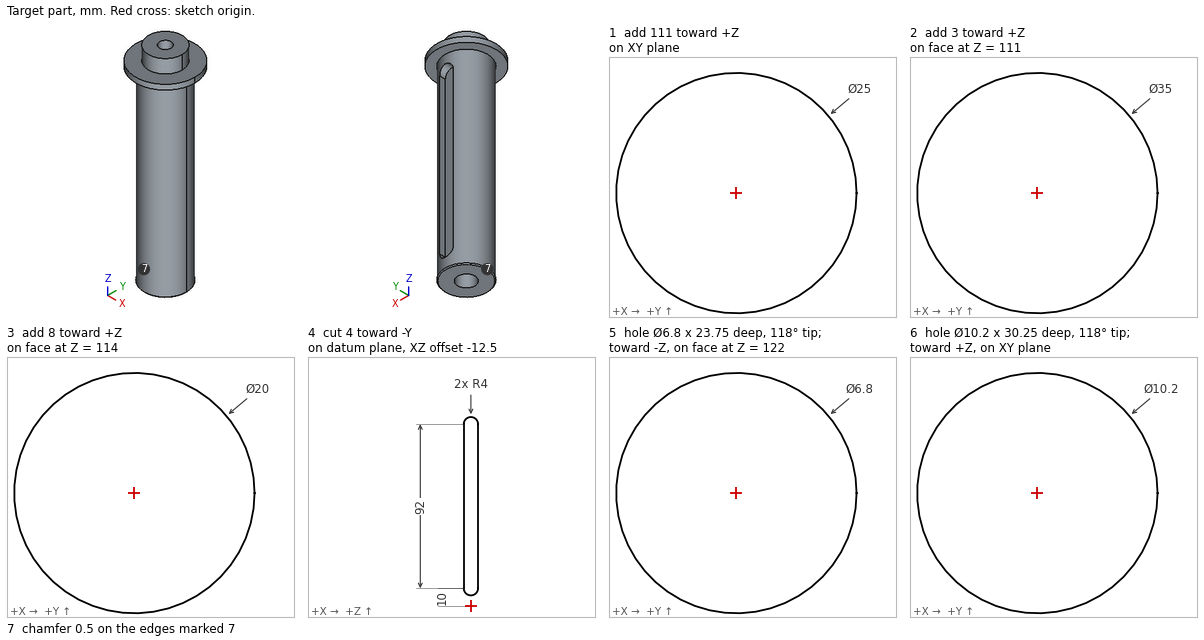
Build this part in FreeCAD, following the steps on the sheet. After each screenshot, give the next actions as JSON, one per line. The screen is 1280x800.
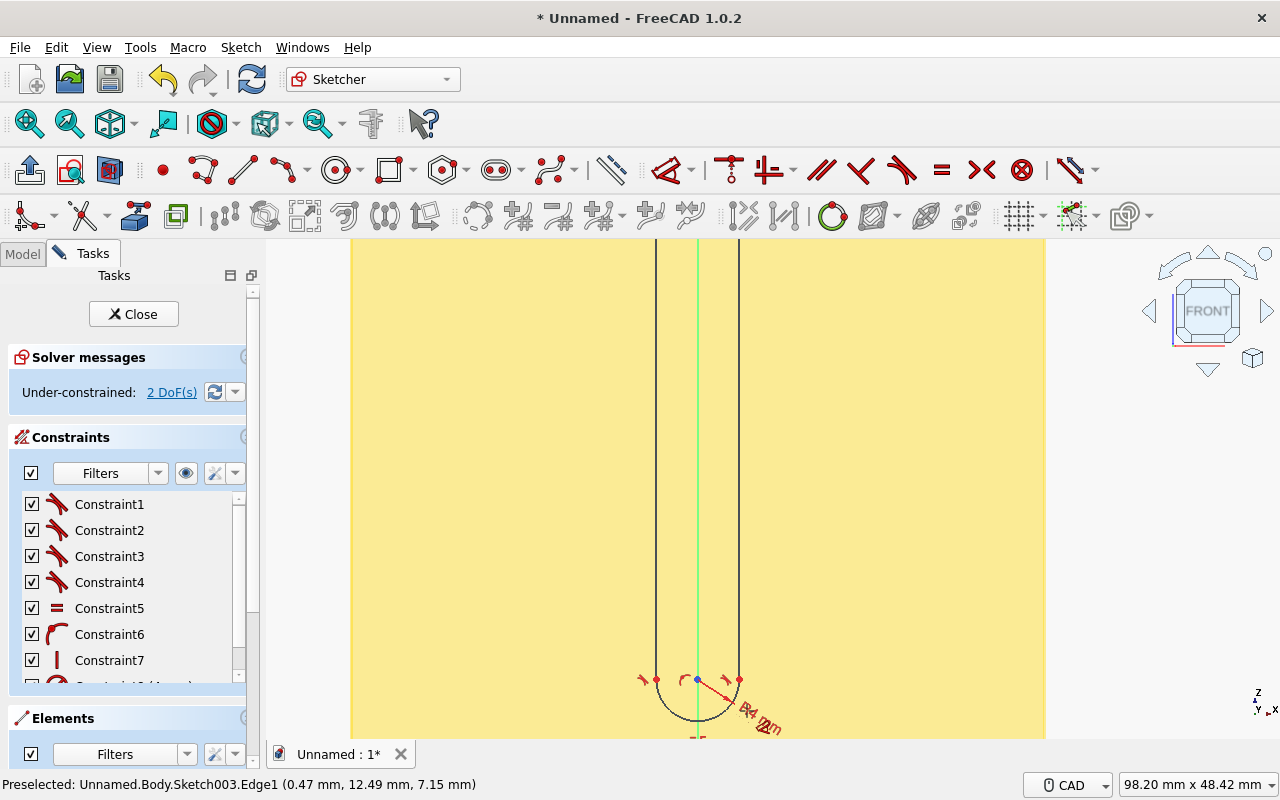
{"action": "left_click", "coordinate": [656, 395]}
{"action": "left_click", "coordinate": [622, 473]}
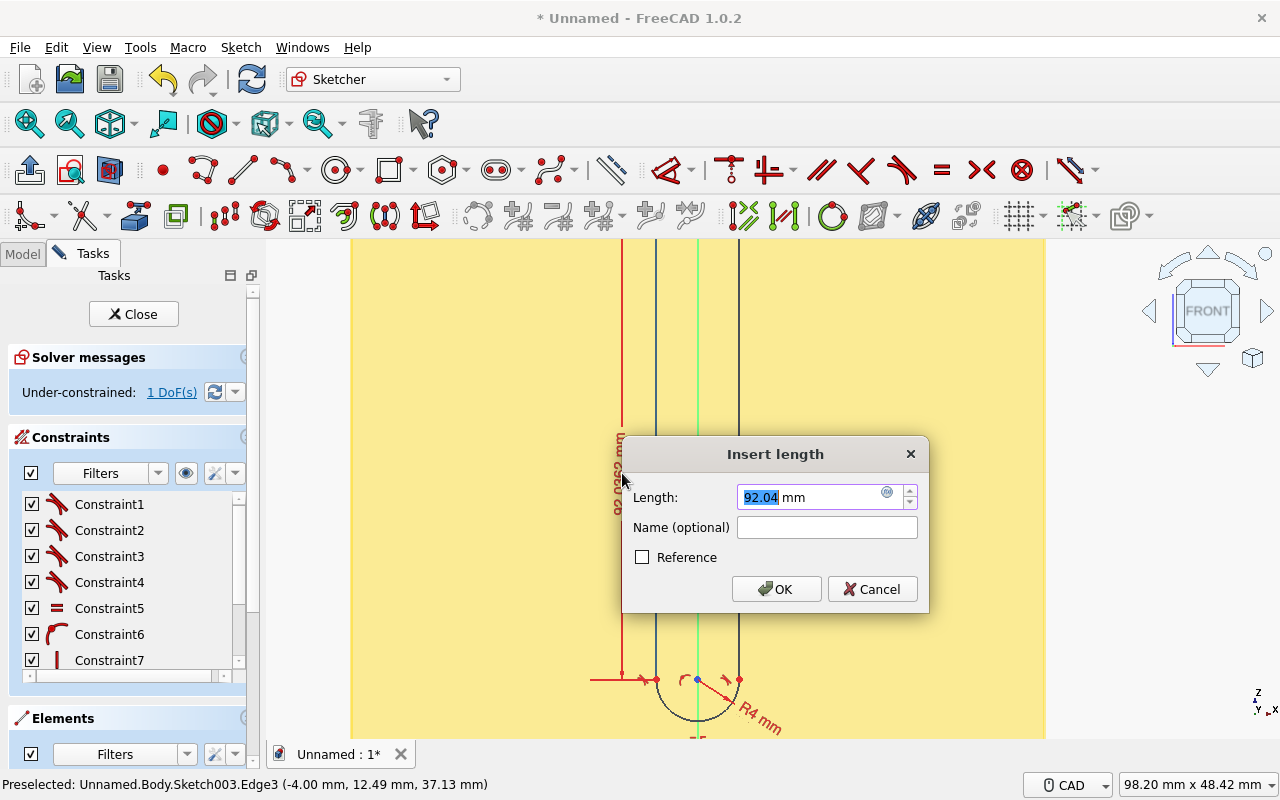
{"action": "type", "text": "92"}
{"action": "key", "text": "Return"}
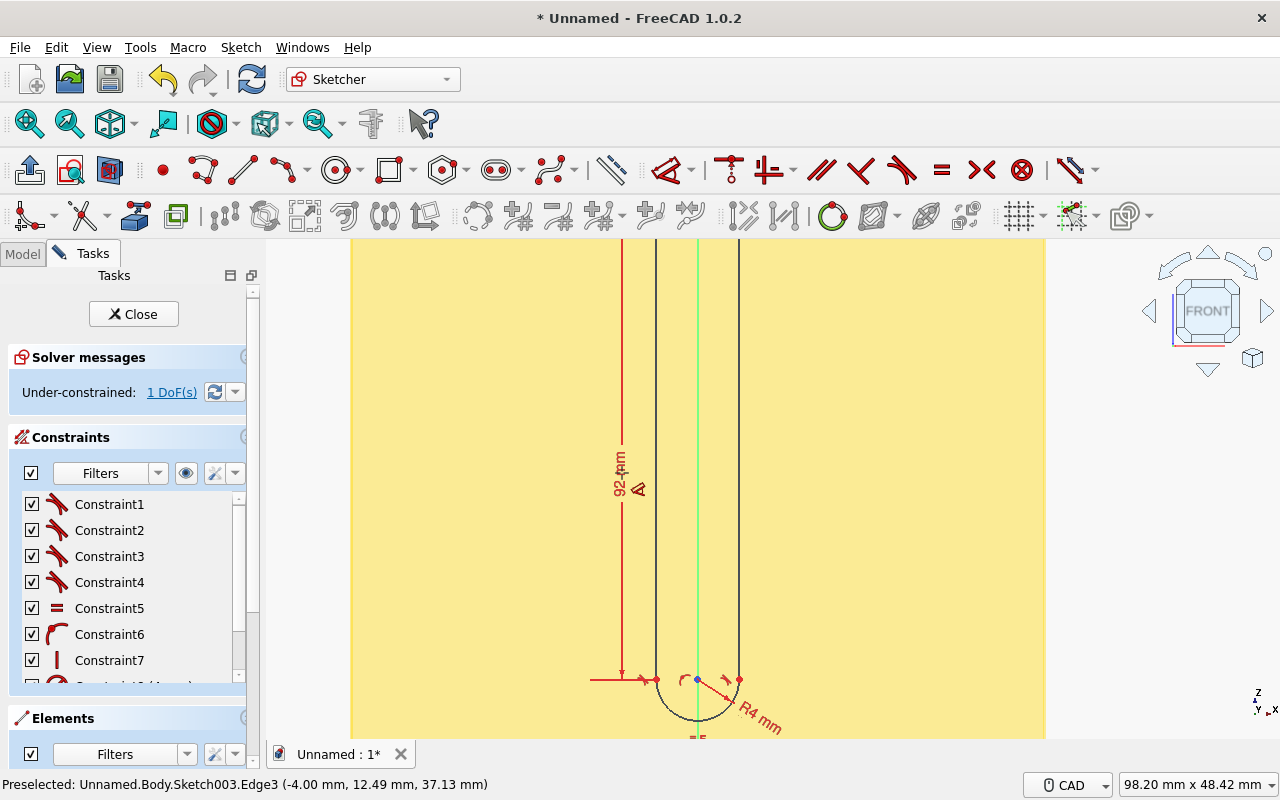
{"action": "left_click", "coordinate": [656, 680]}
{"action": "left_click", "coordinate": [622, 695]}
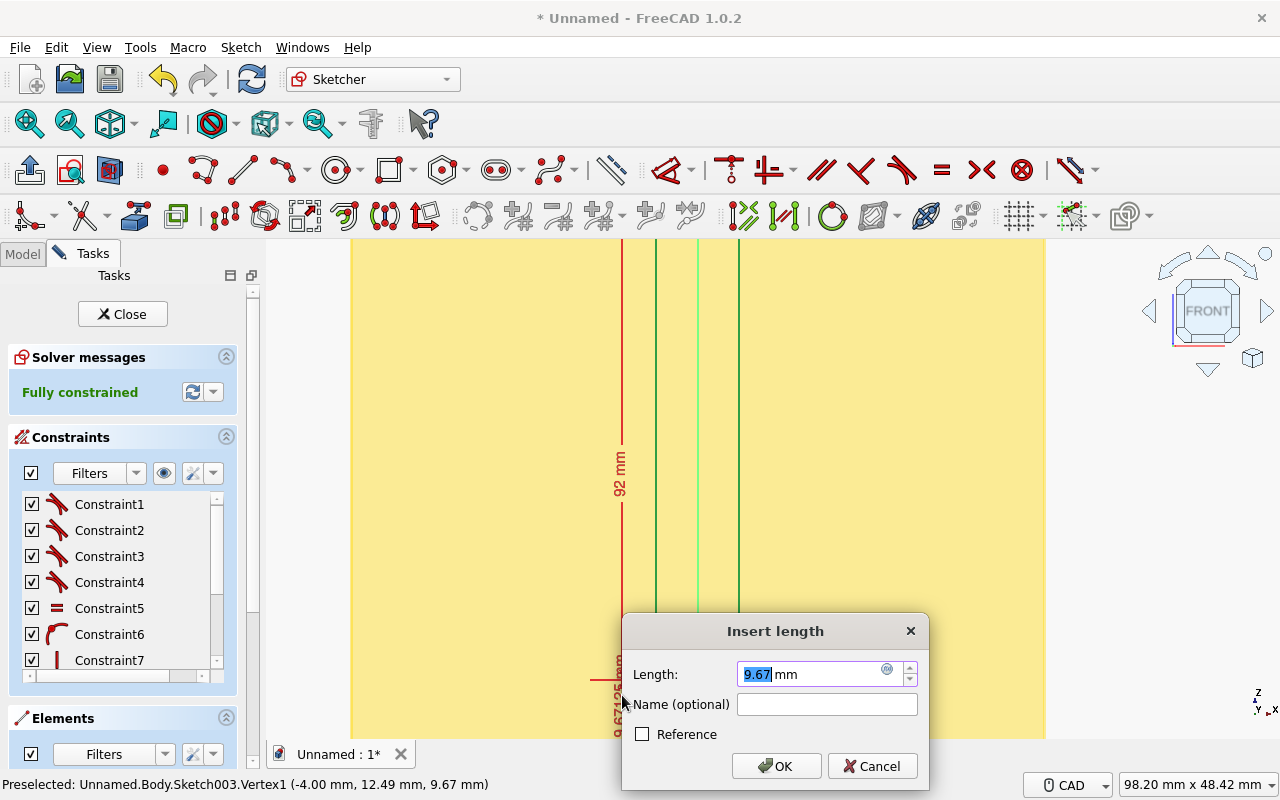
{"action": "type", "text": "10"}
{"action": "key", "text": "Return"}
{"action": "key", "text": "Escape"}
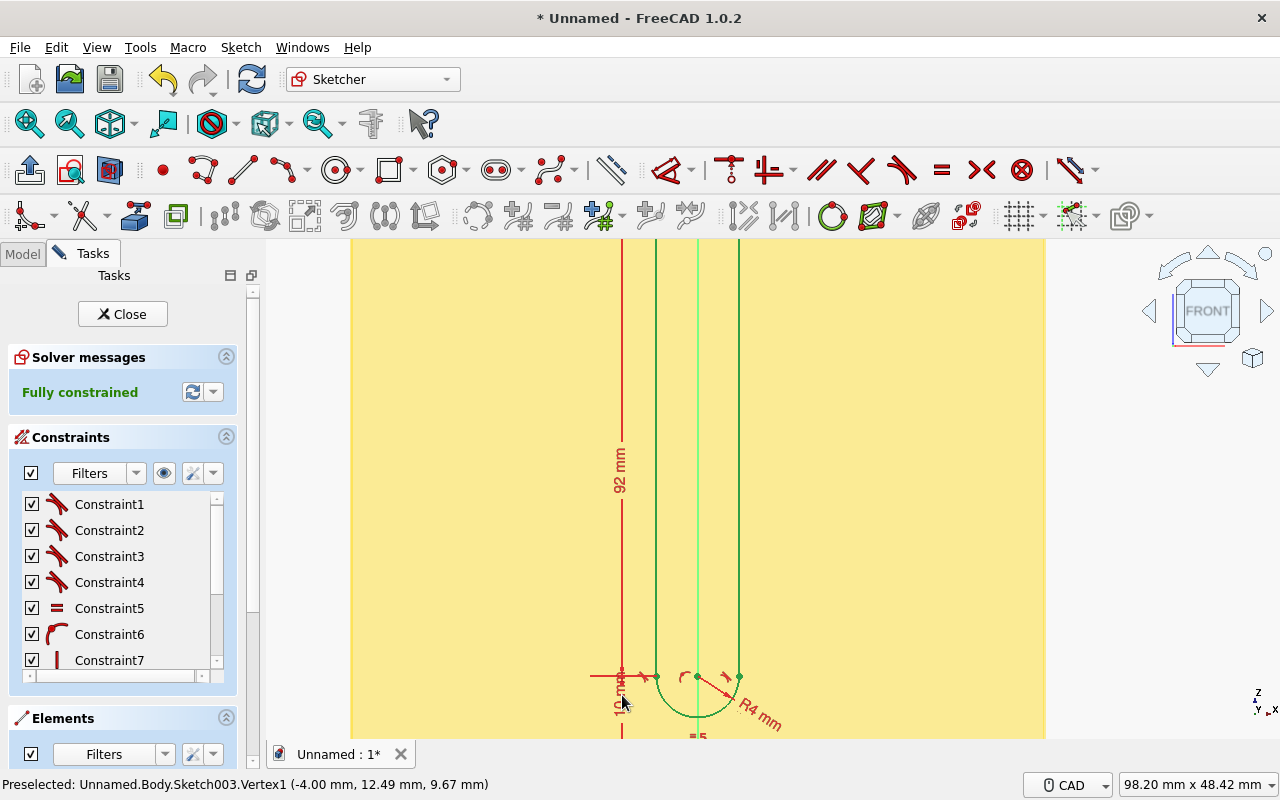
{"action": "left_click", "coordinate": [123, 314]}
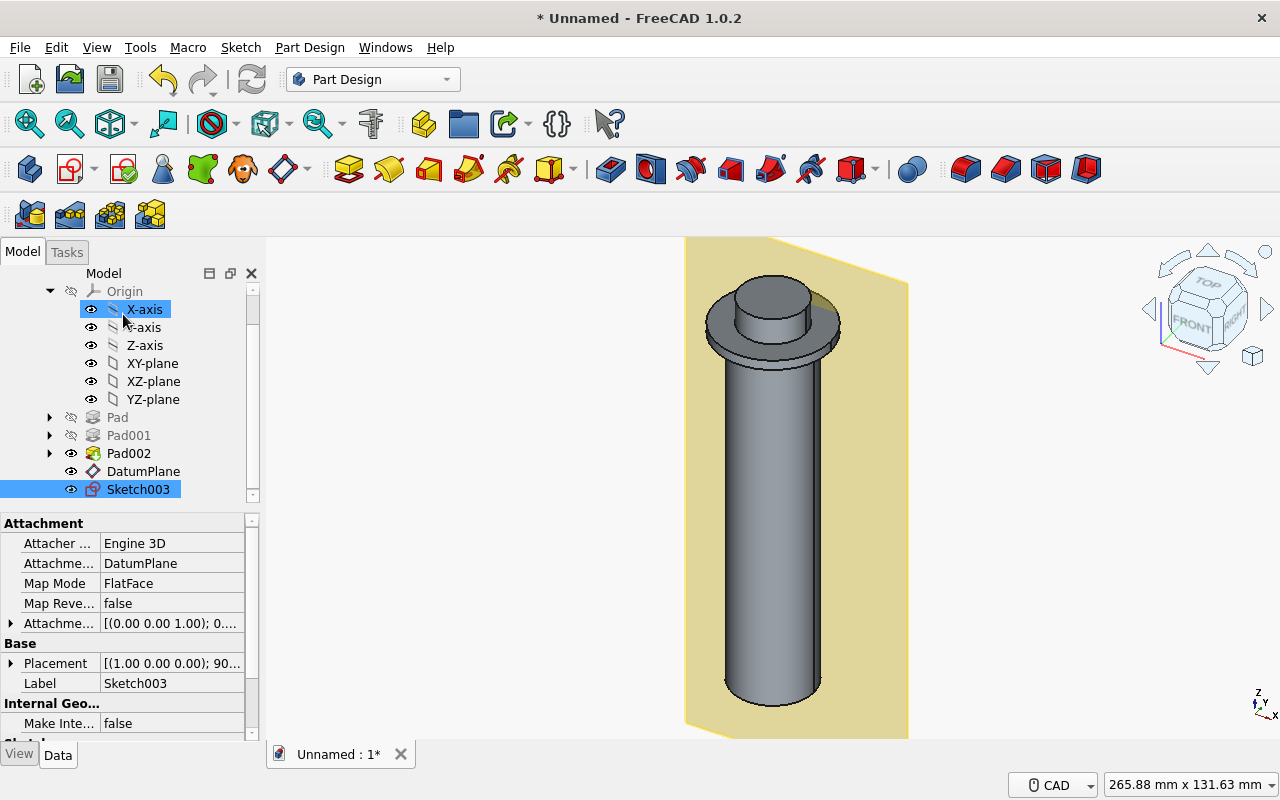
{"action": "left_click", "coordinate": [612, 170]}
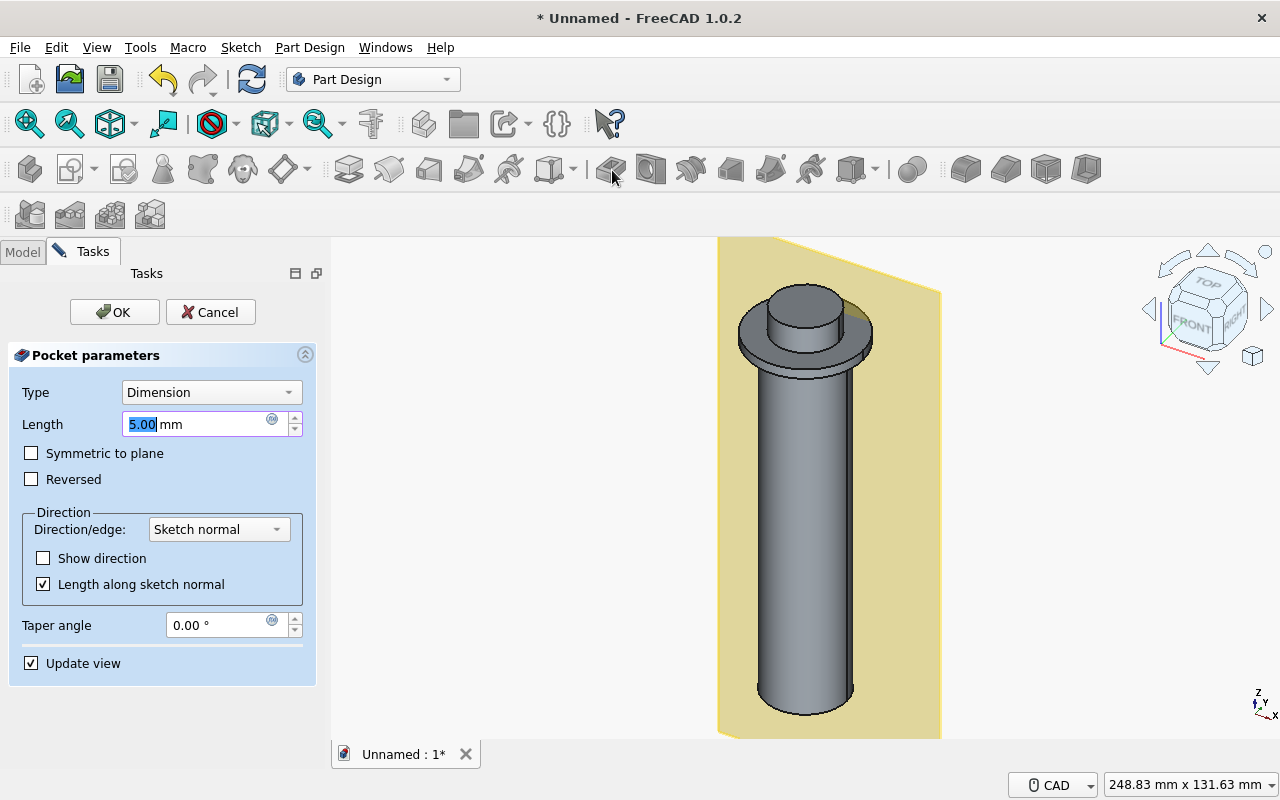
{"action": "type", "text": "4"}
{"action": "key", "text": "Tab"}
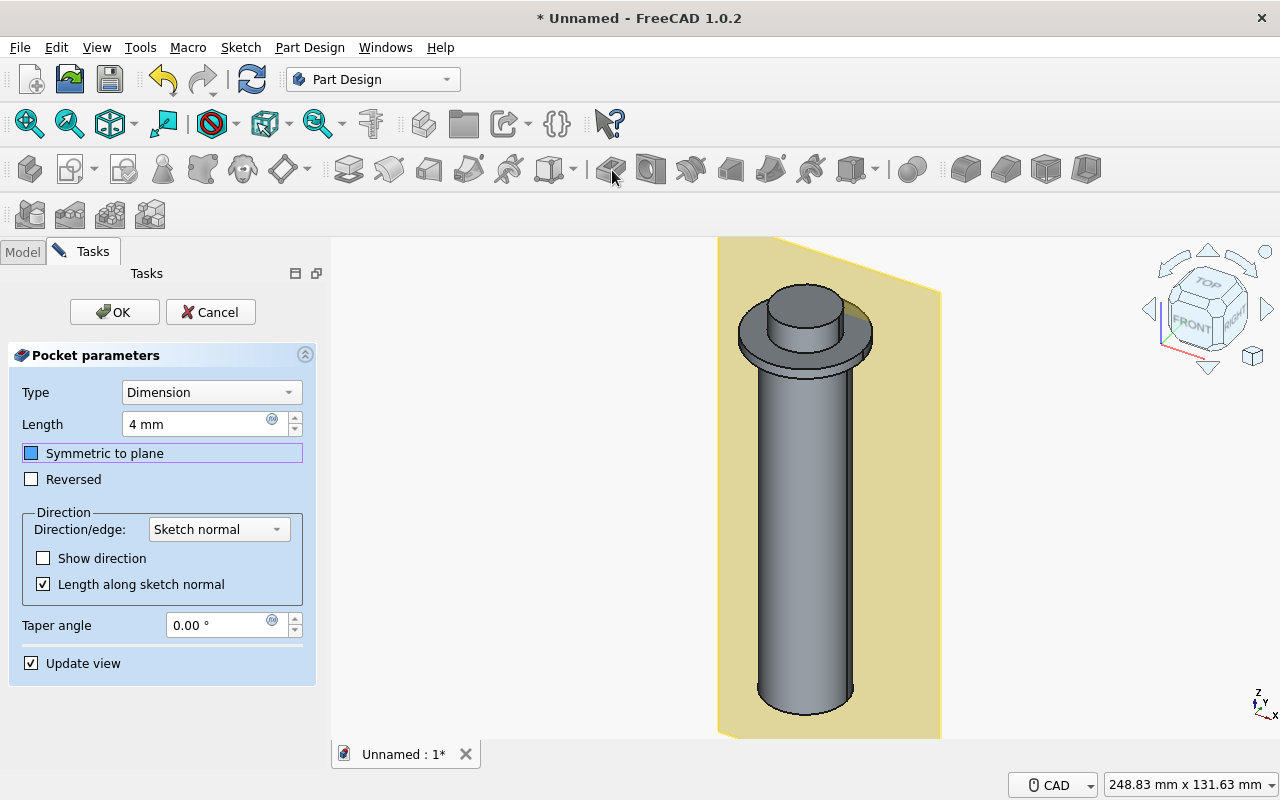
{"action": "left_click", "coordinate": [30, 479]}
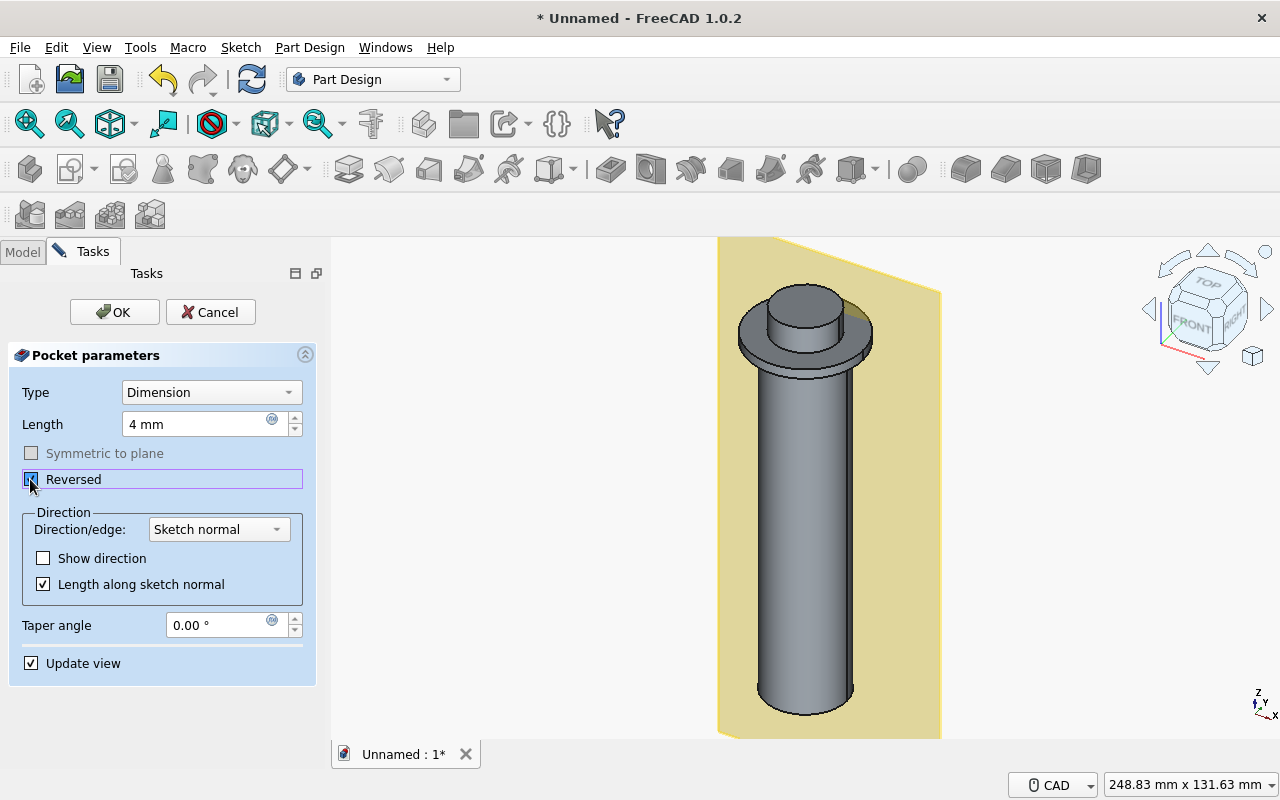
{"action": "left_click", "coordinate": [115, 312]}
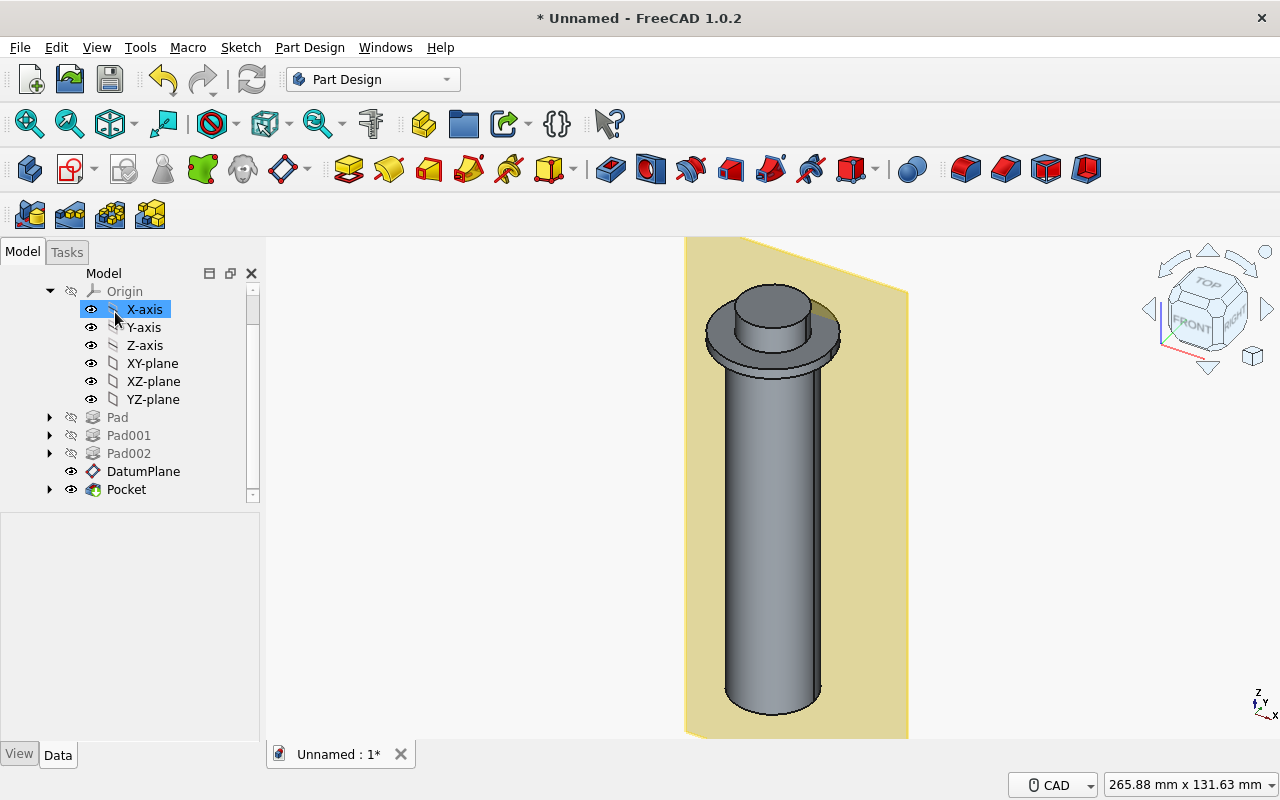
{"action": "left_click", "coordinate": [116, 471]}
{"action": "key", "text": "space"}